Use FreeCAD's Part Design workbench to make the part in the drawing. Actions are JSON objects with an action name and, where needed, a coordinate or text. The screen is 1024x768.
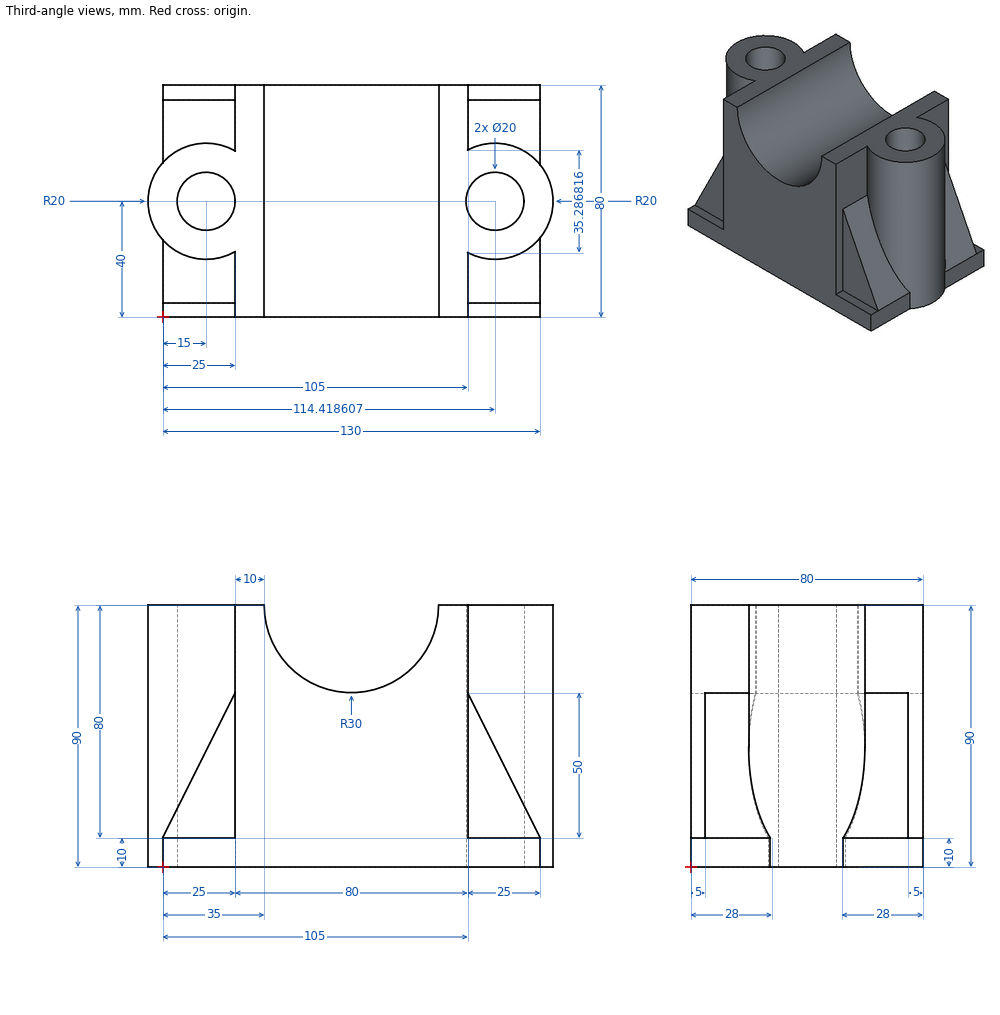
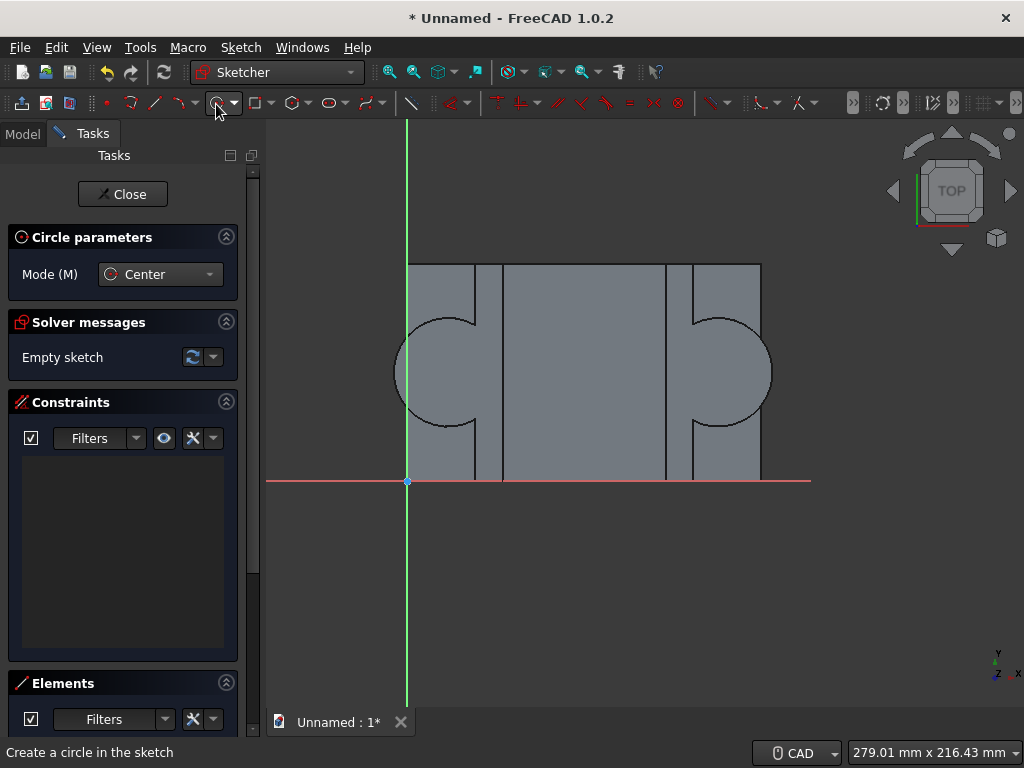
{"action": "left_click", "coordinate": [718, 372]}
{"action": "left_click", "coordinate": [737, 353]}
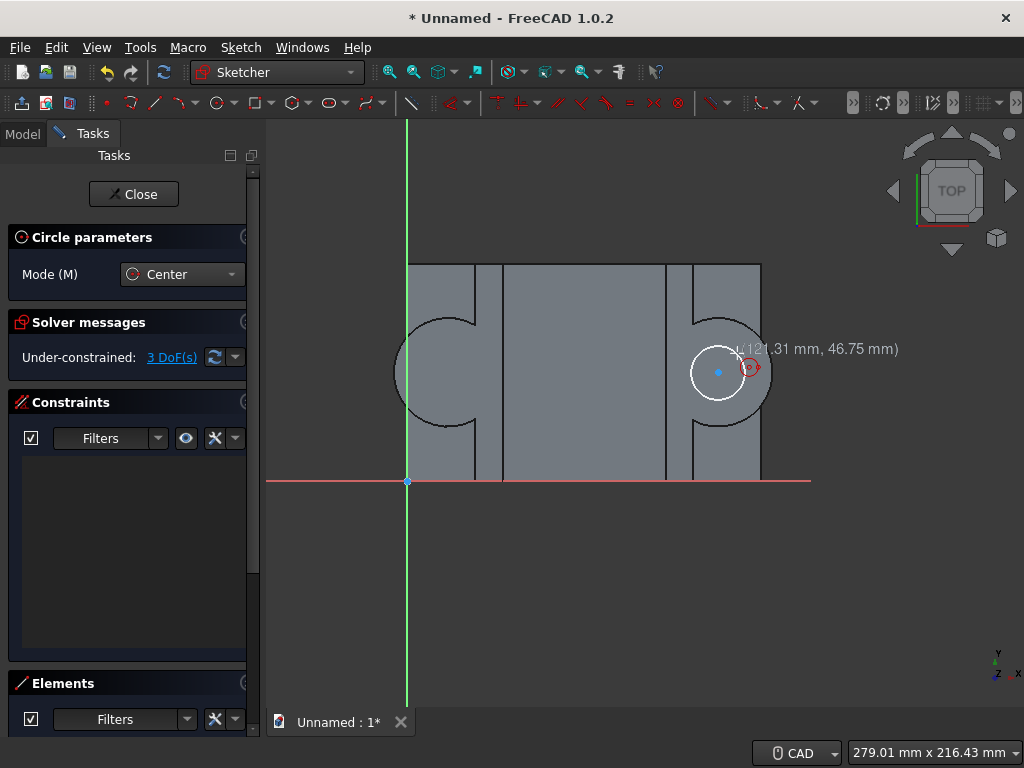
{"action": "left_click", "coordinate": [448, 372]}
{"action": "left_click", "coordinate": [467, 353]}
{"action": "key", "text": "Escape"}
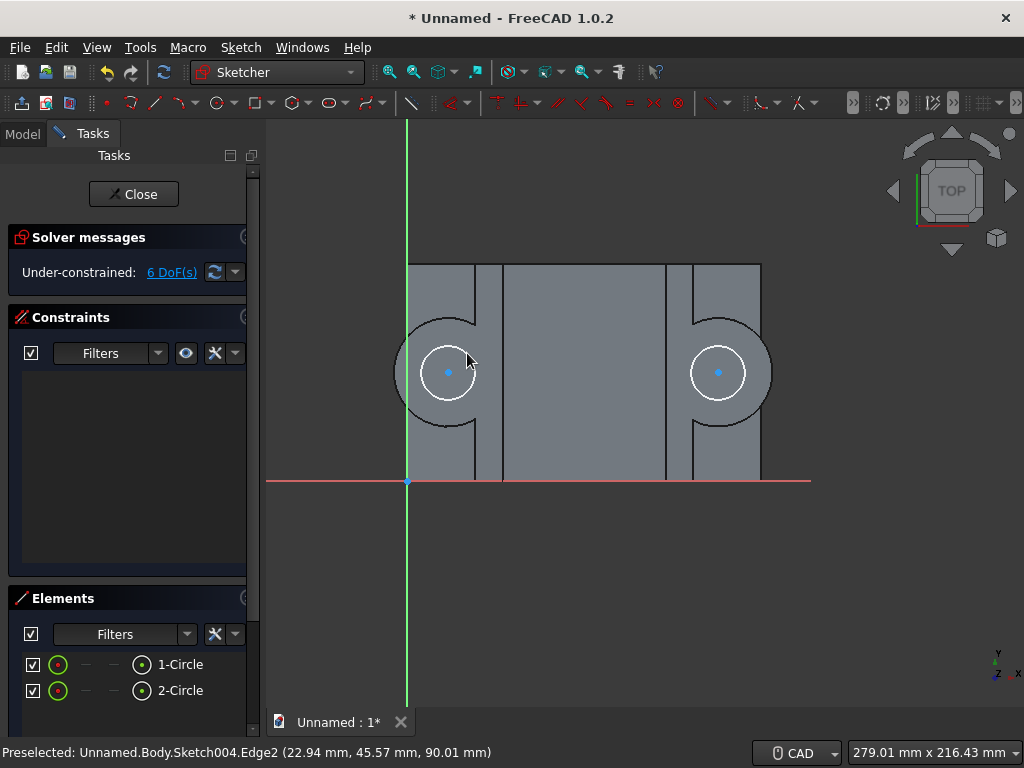
{"action": "left_click", "coordinate": [737, 354]}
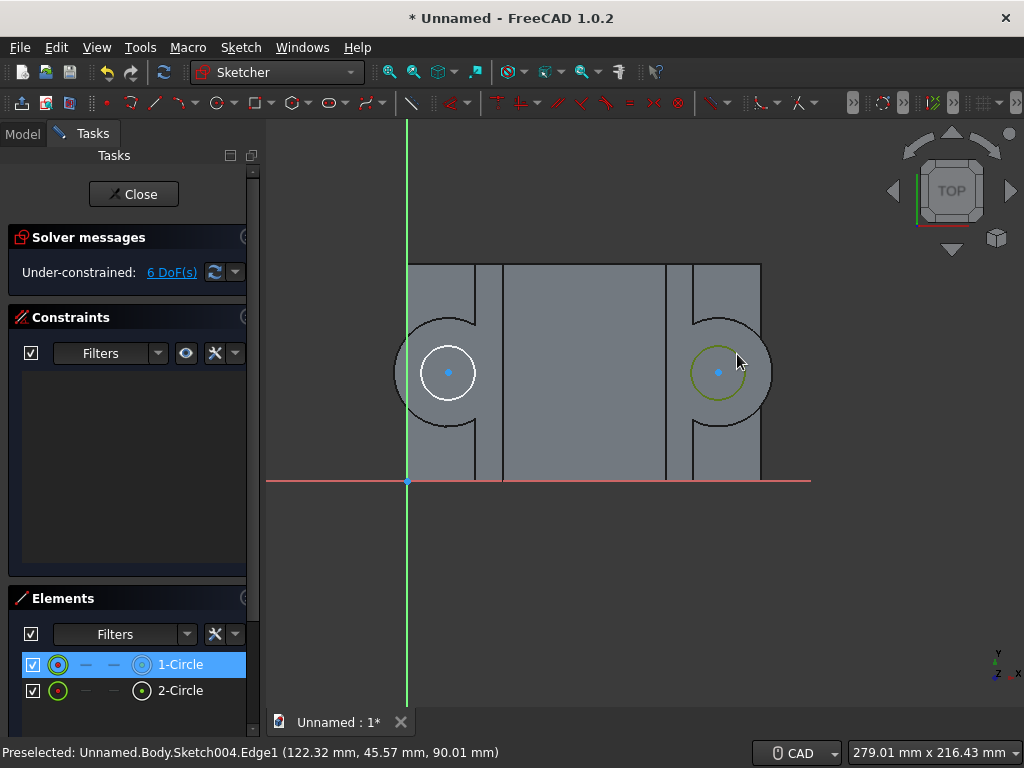
{"action": "left_click", "coordinate": [467, 354]}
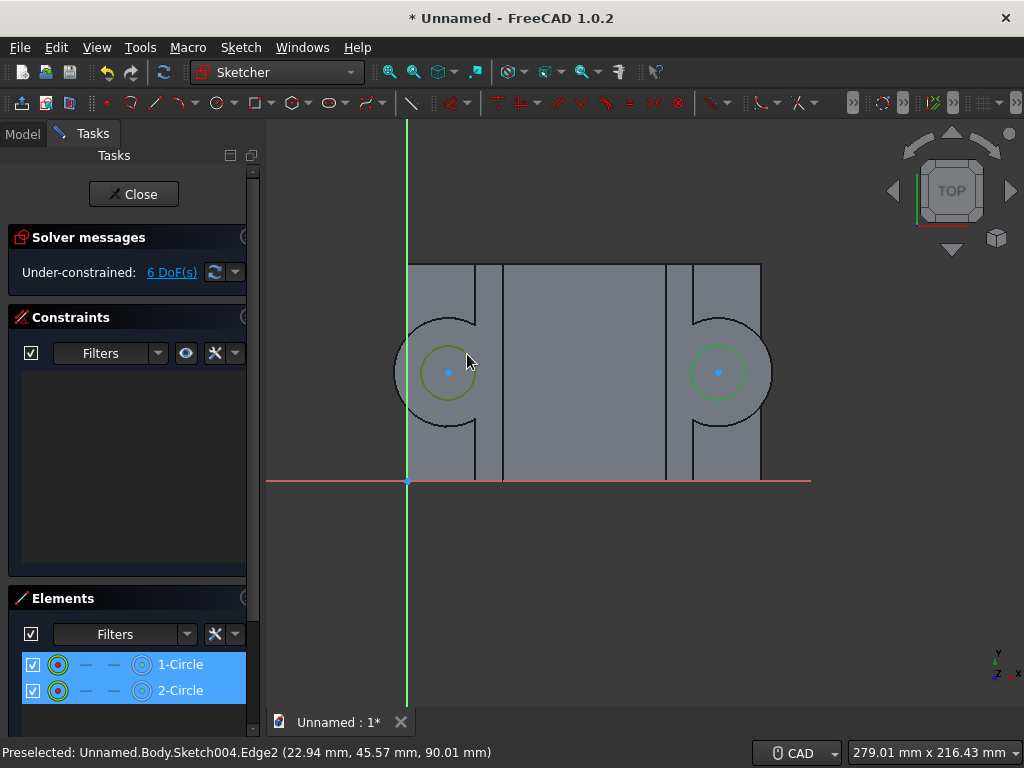
{"action": "left_click", "coordinate": [630, 104]}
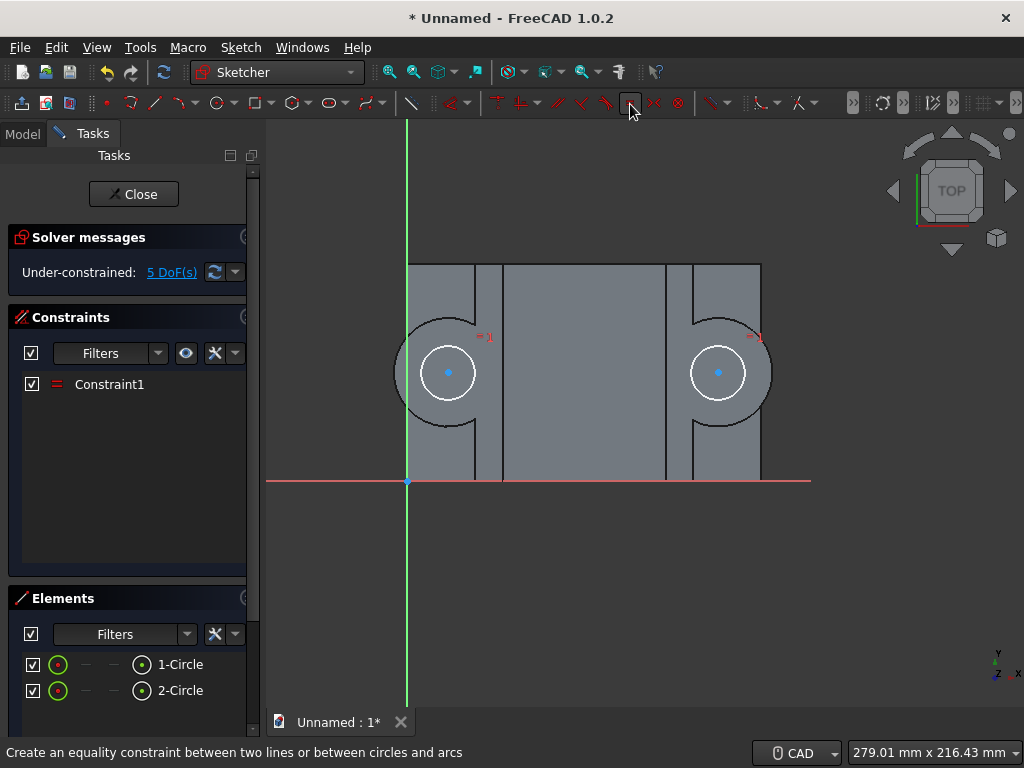
{"action": "left_click", "coordinate": [450, 104]}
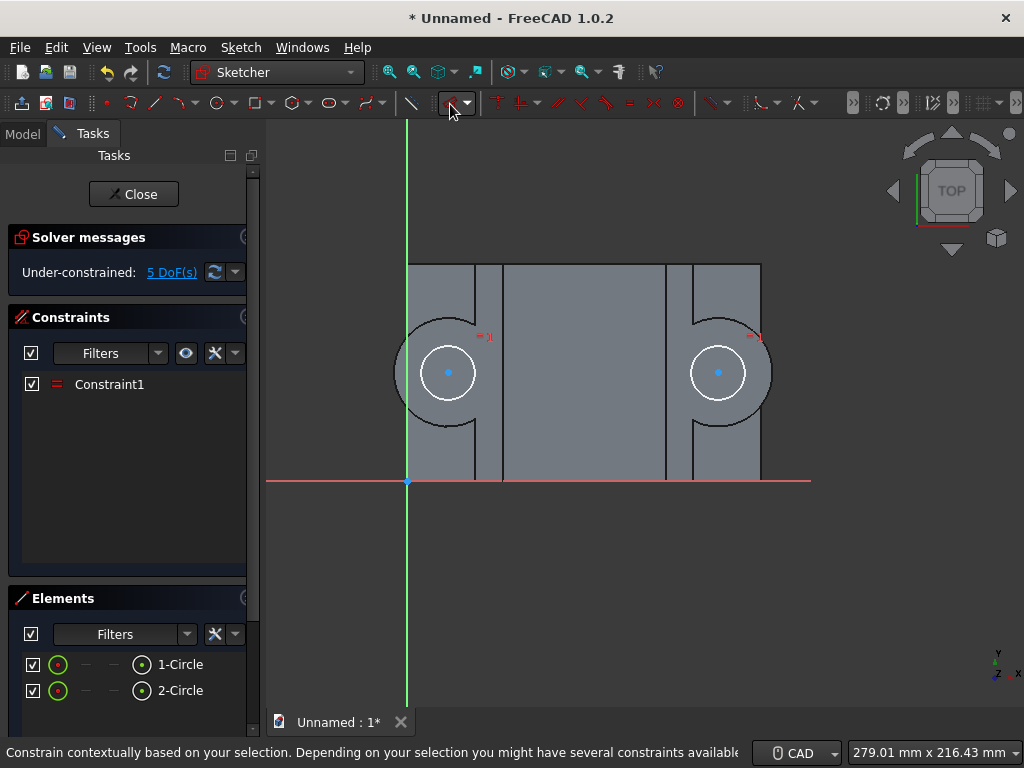
{"action": "left_click", "coordinate": [737, 354]}
{"action": "left_click", "coordinate": [760, 331]}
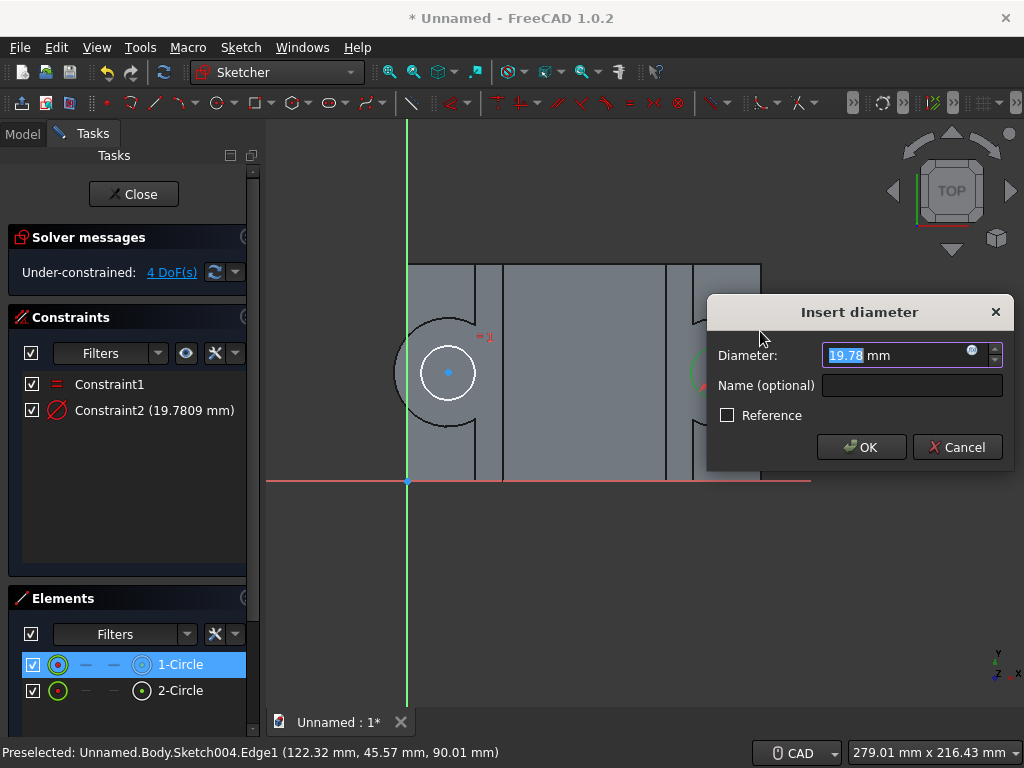
{"action": "type", "text": "20"}
{"action": "key", "text": "Return"}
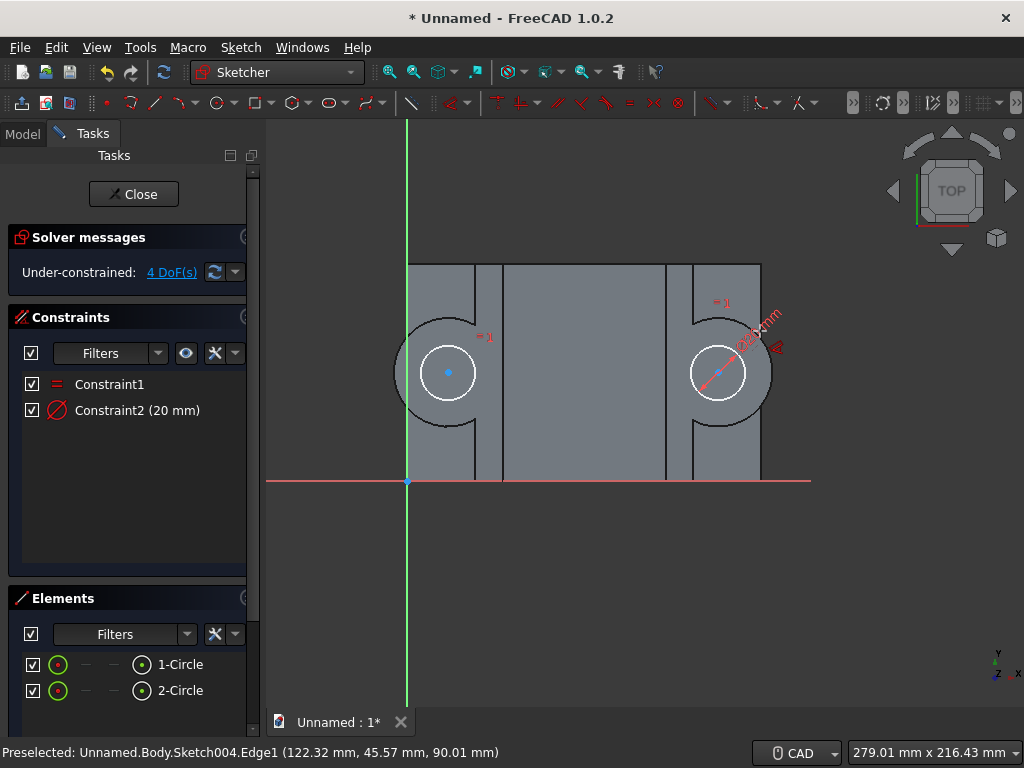
{"action": "left_click", "coordinate": [718, 373]}
{"action": "left_click", "coordinate": [373, 427]}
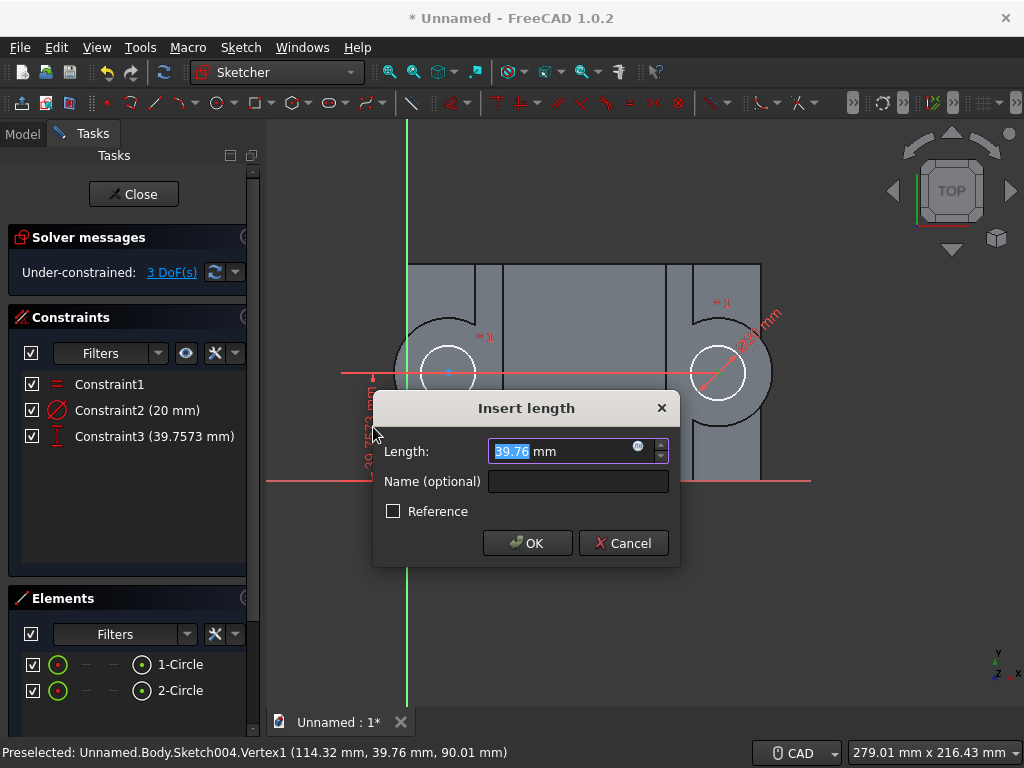
{"action": "type", "text": "40"}
{"action": "key", "text": "Return"}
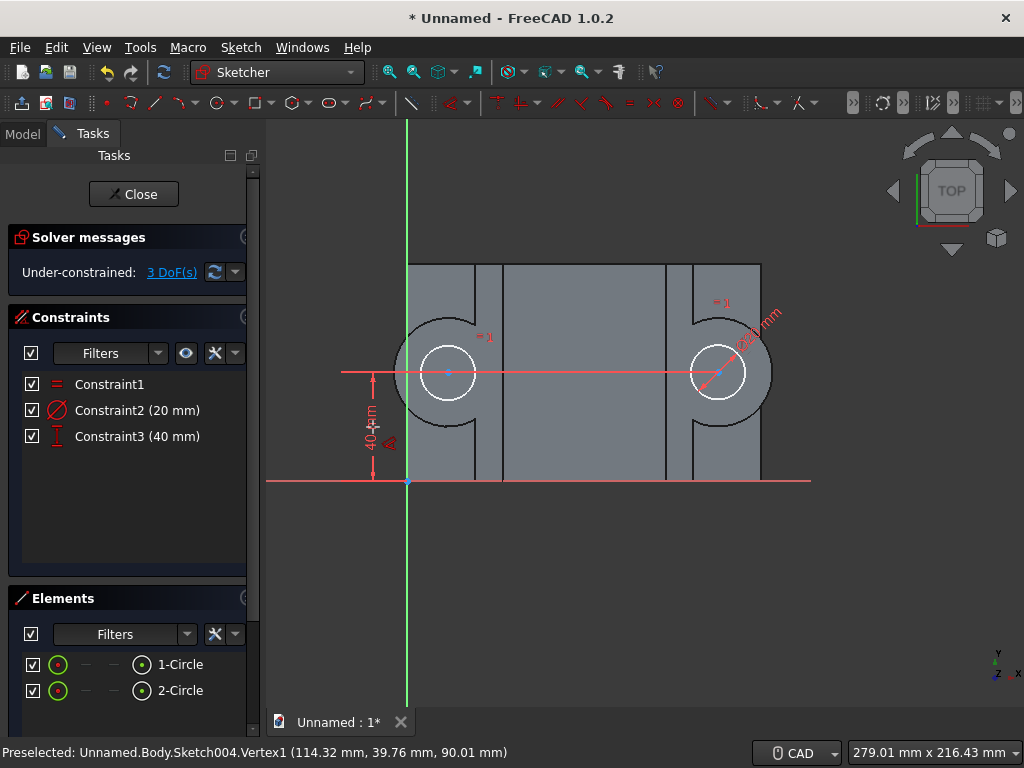
{"action": "left_click", "coordinate": [448, 373]}
{"action": "left_click", "coordinate": [428, 515]}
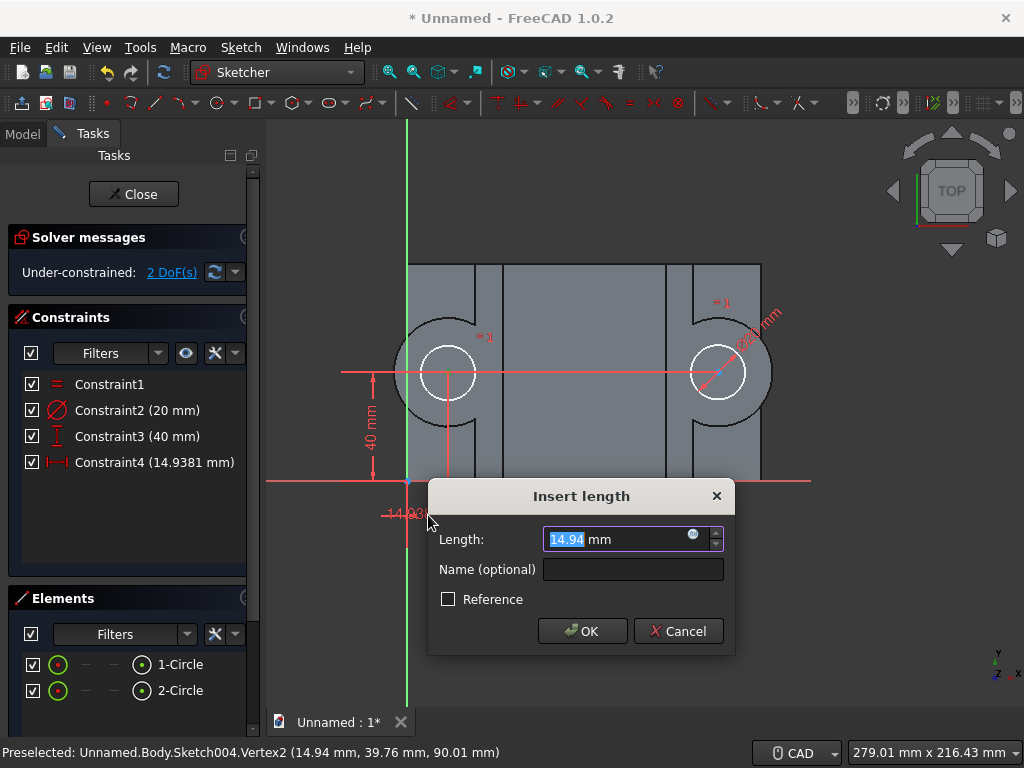
{"action": "type", "text": "15"}
{"action": "key", "text": "Return"}